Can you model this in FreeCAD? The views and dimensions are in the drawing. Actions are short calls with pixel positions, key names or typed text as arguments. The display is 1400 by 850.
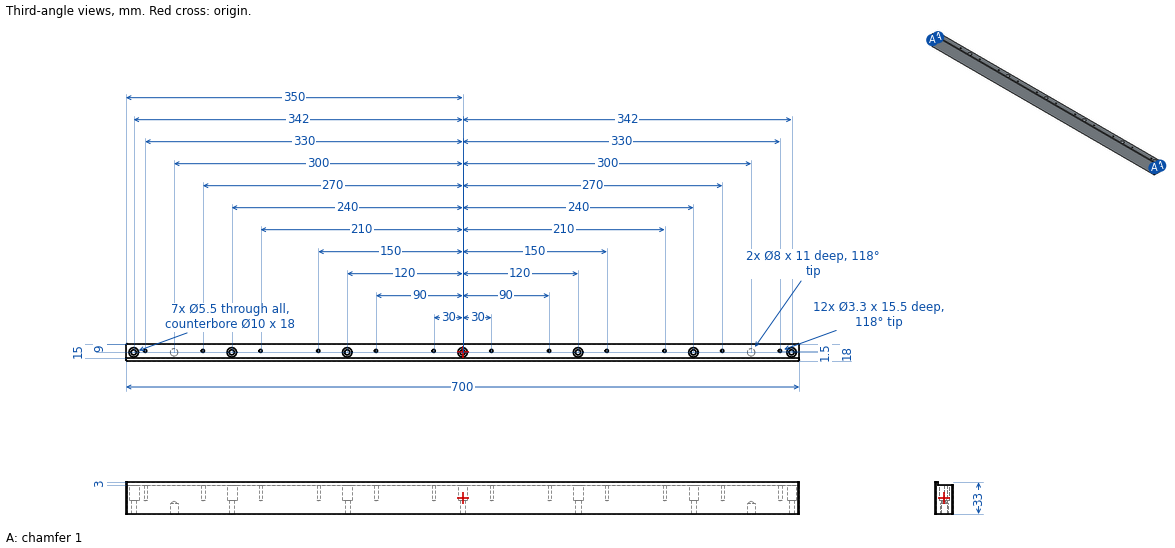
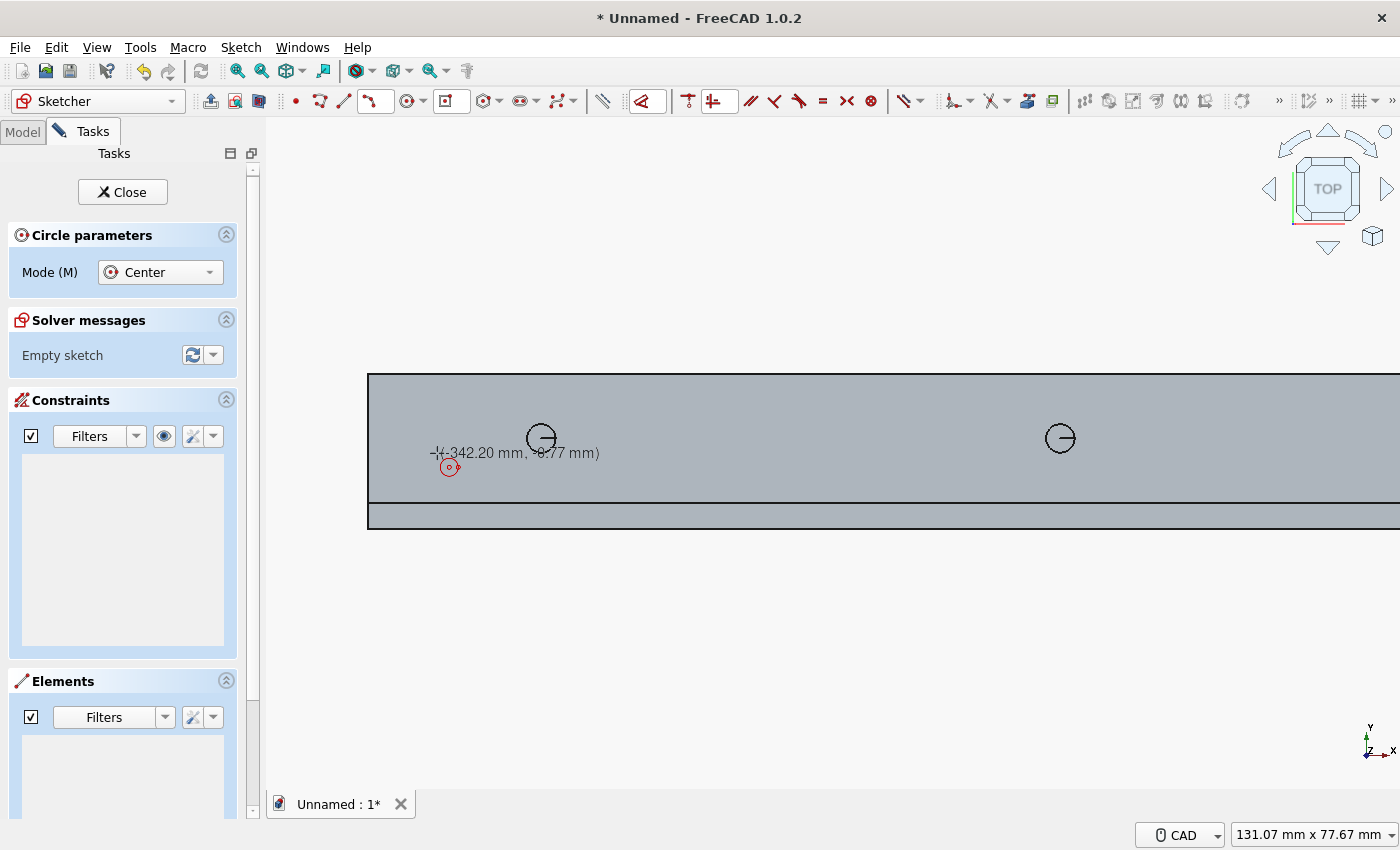
scroll(437, 453, down, 11)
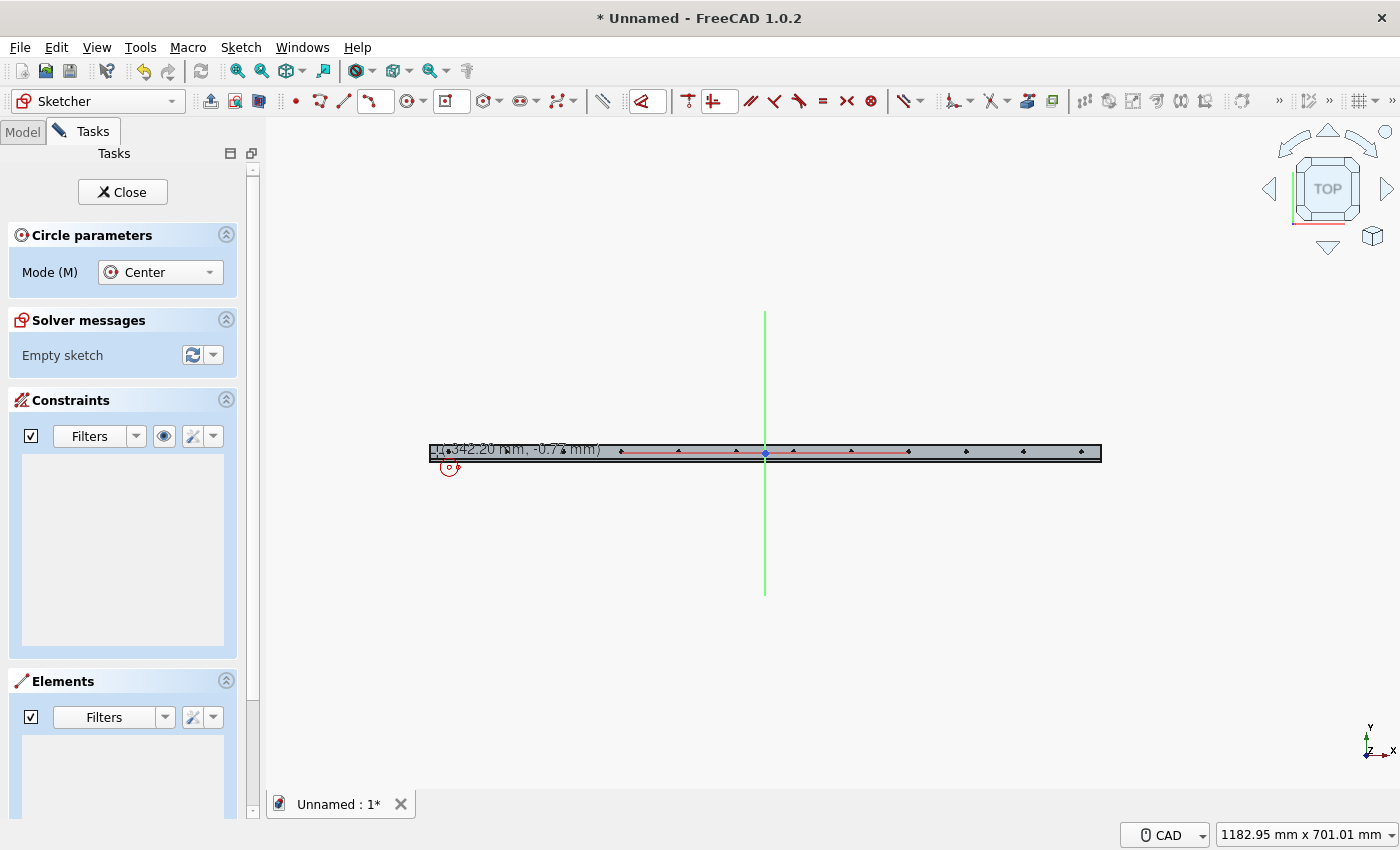
click(437, 453)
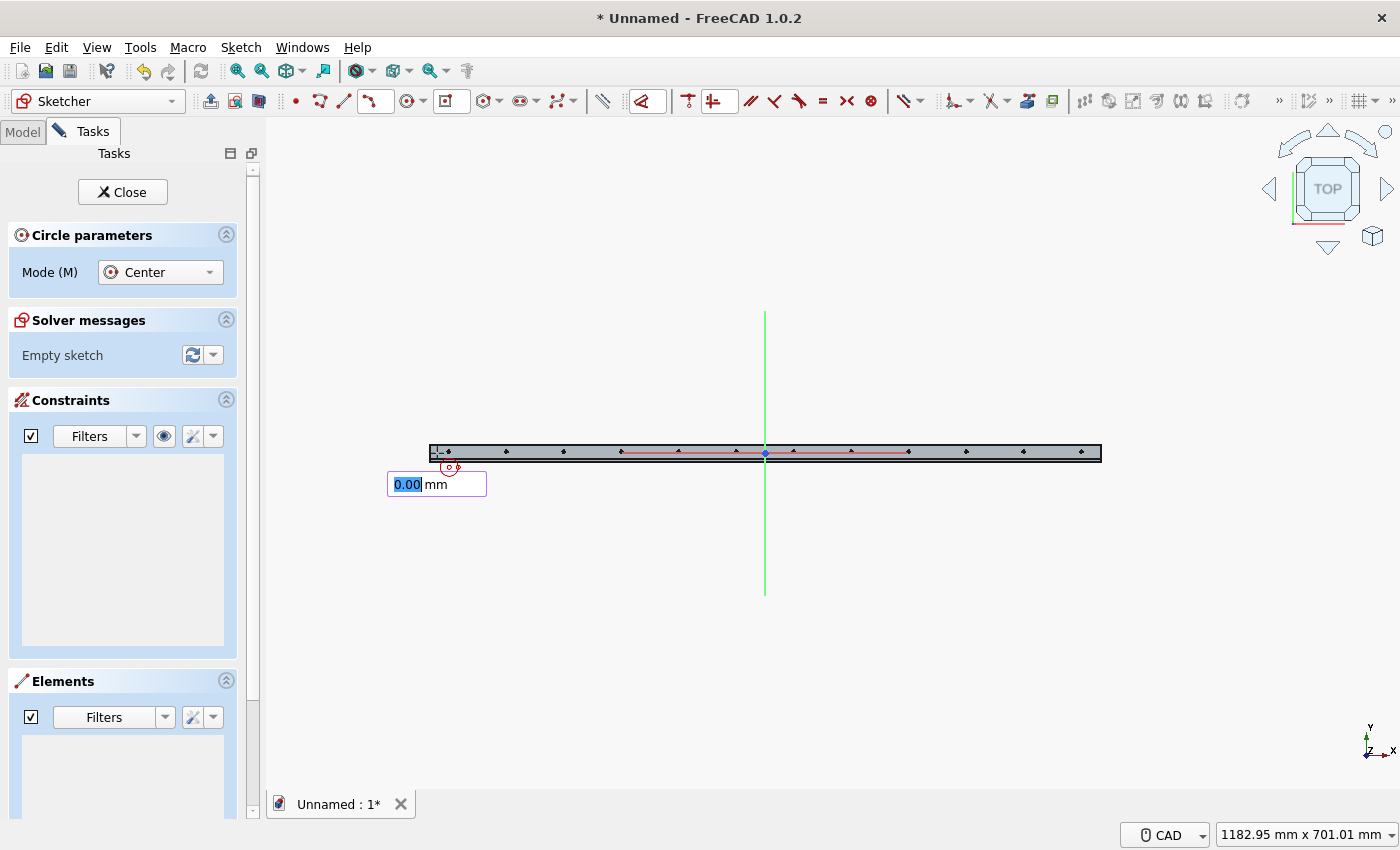
scroll(438, 451, up, 10)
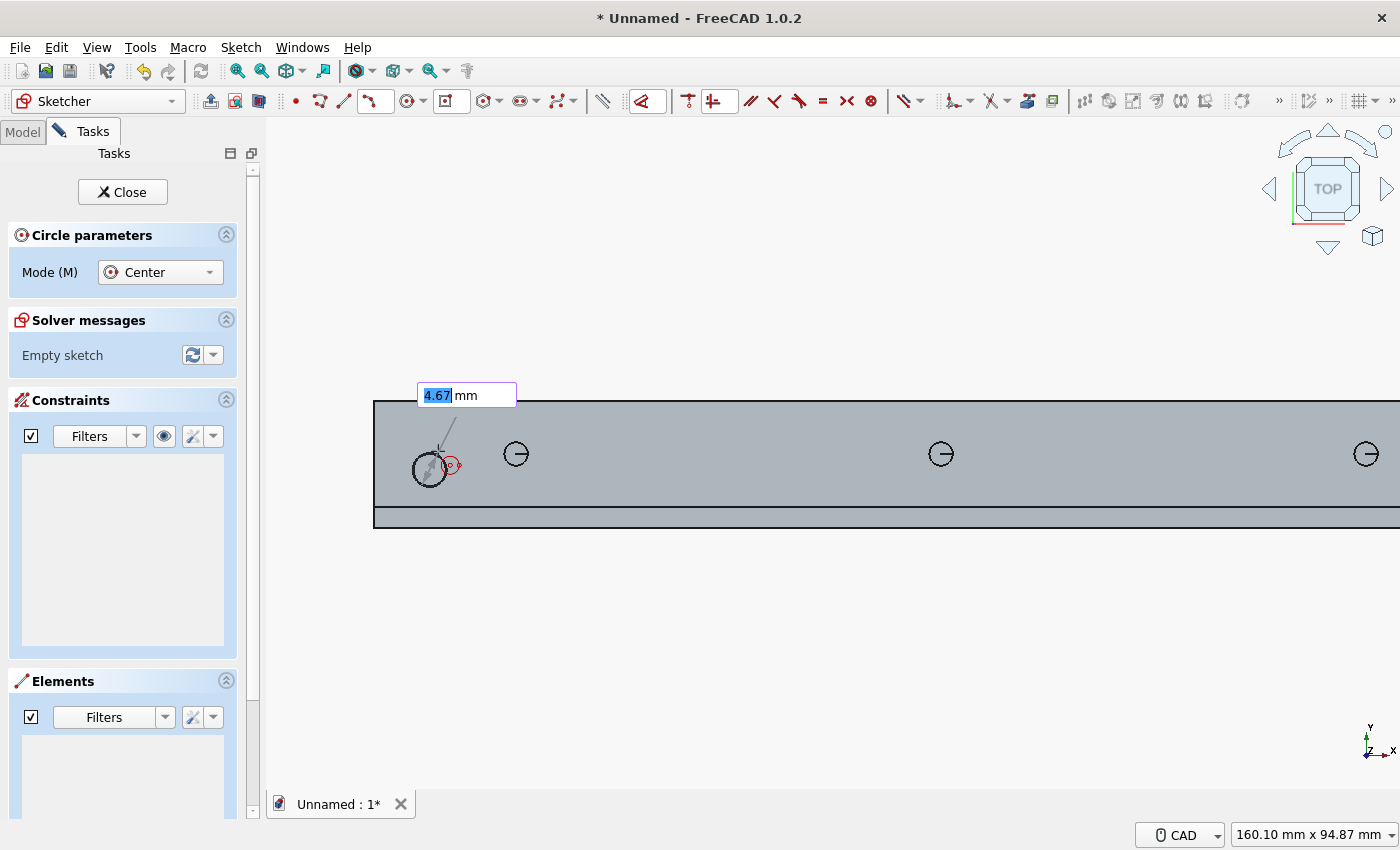
click(438, 446)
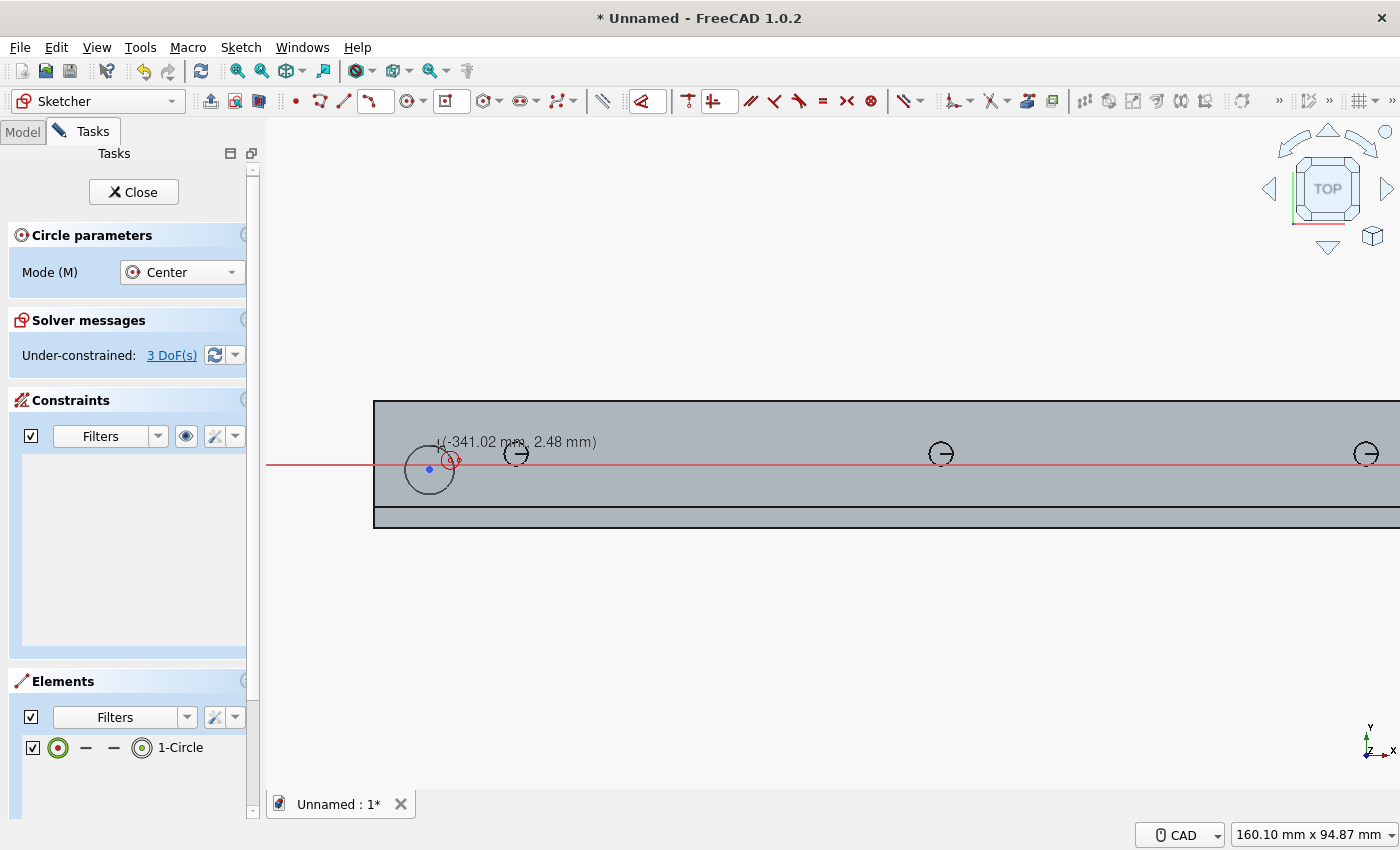
scroll(438, 451, down, 10)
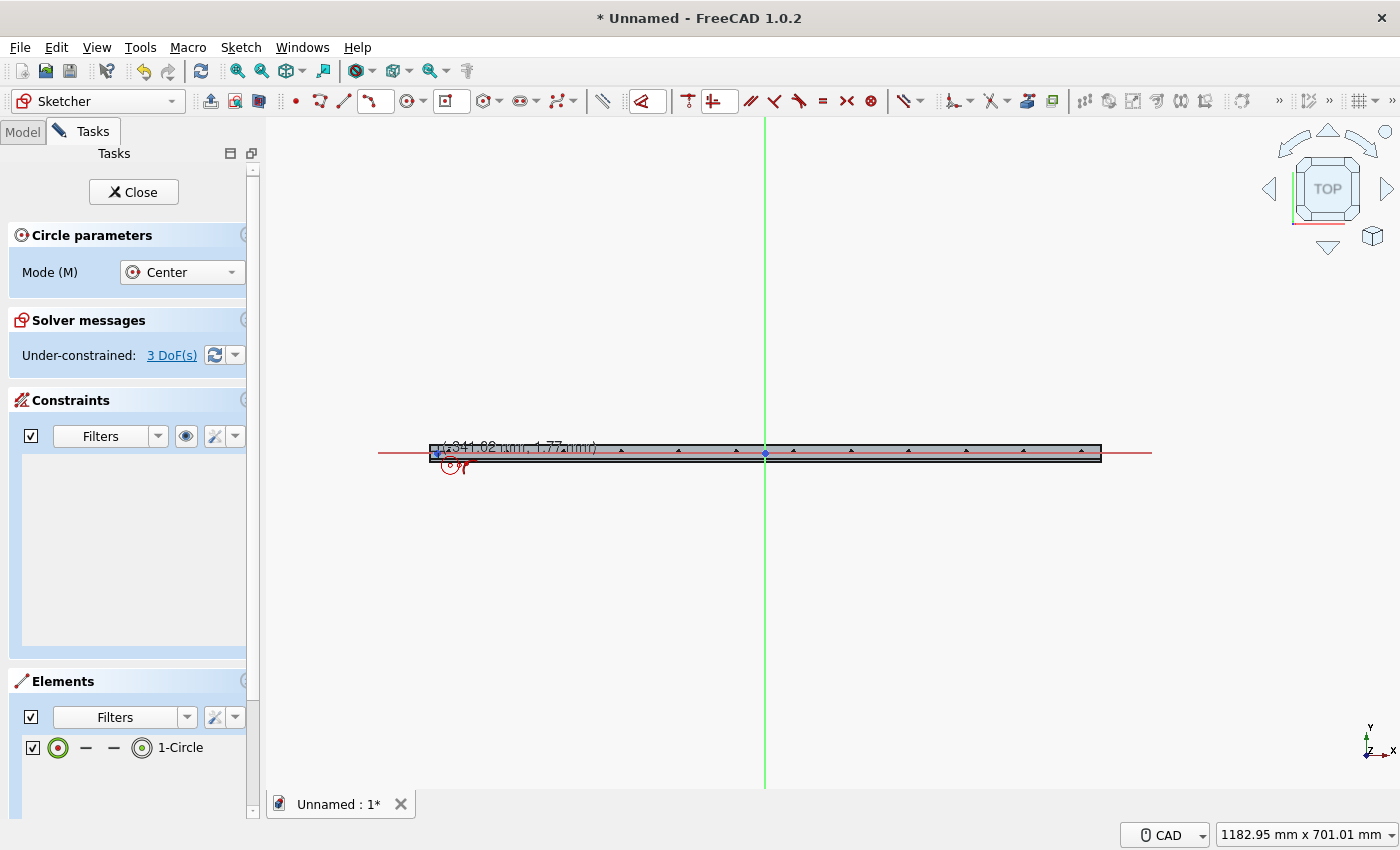
click(535, 453)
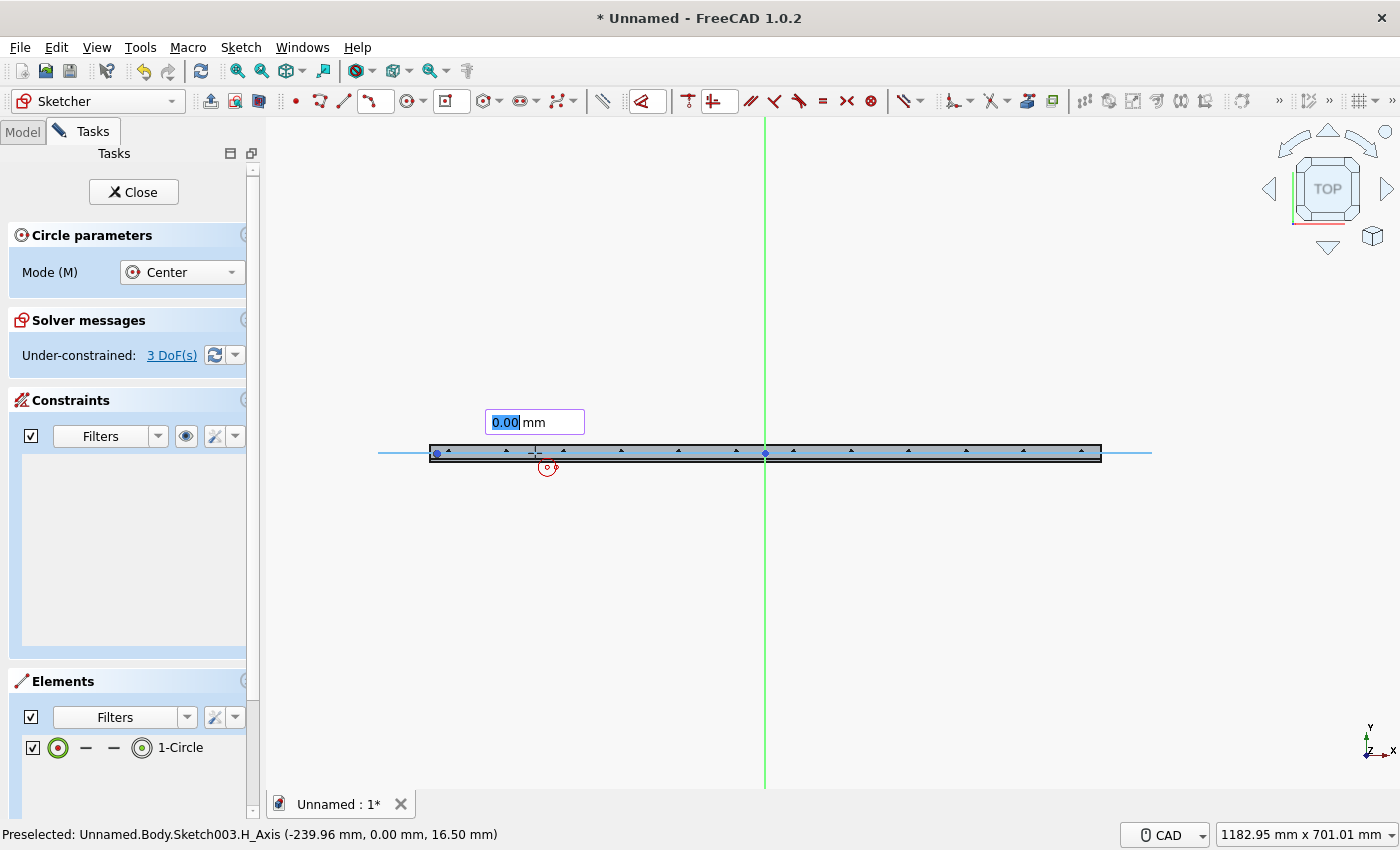
scroll(536, 451, up, 10)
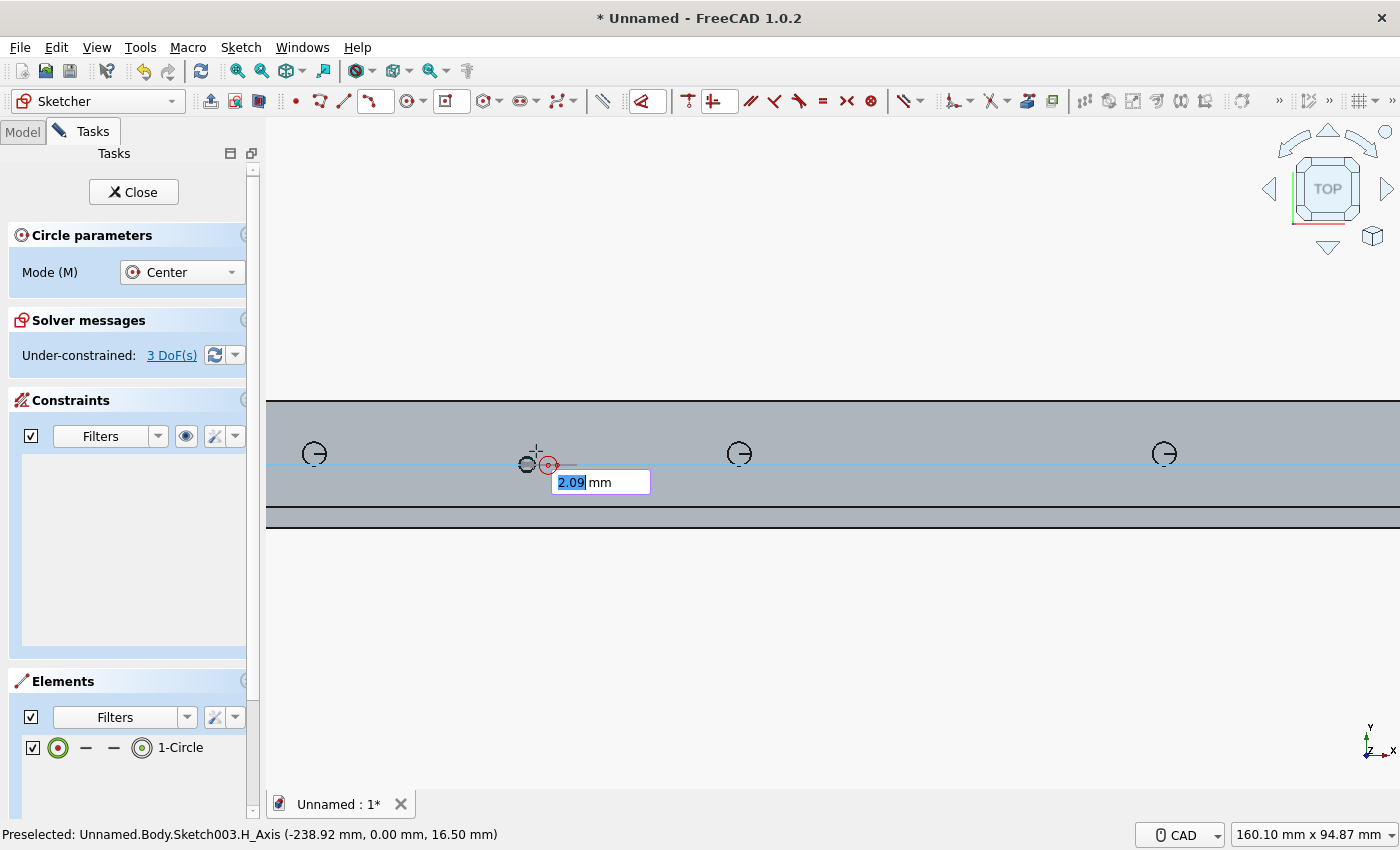
click(534, 446)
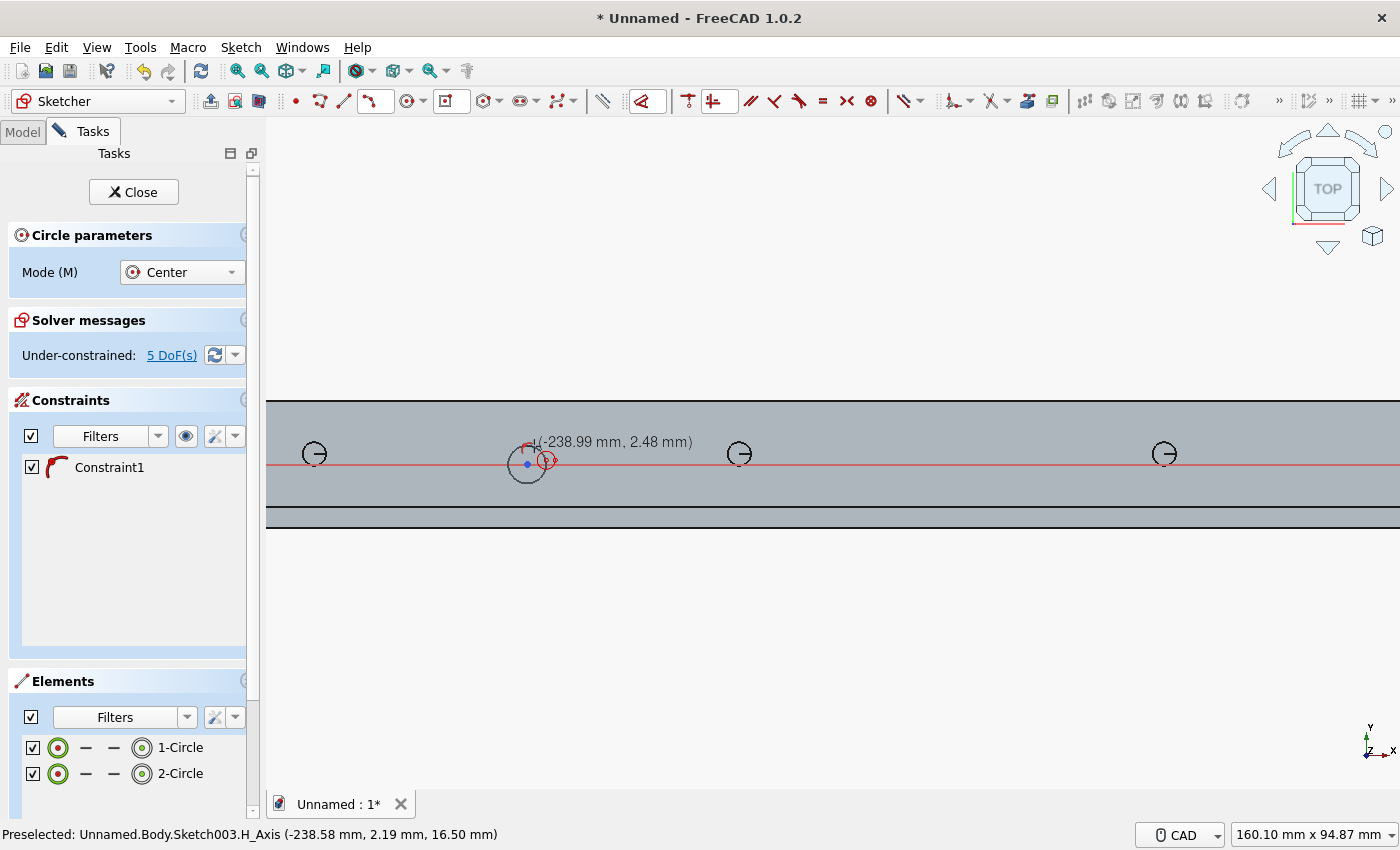
scroll(536, 451, down, 10)